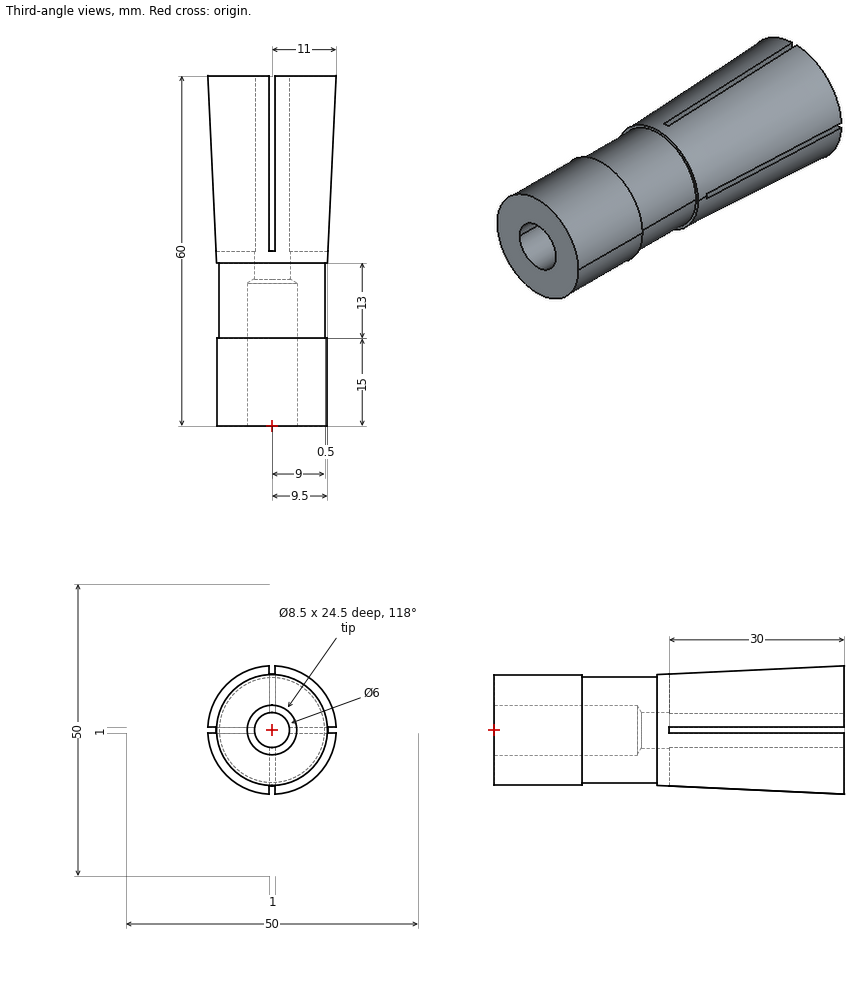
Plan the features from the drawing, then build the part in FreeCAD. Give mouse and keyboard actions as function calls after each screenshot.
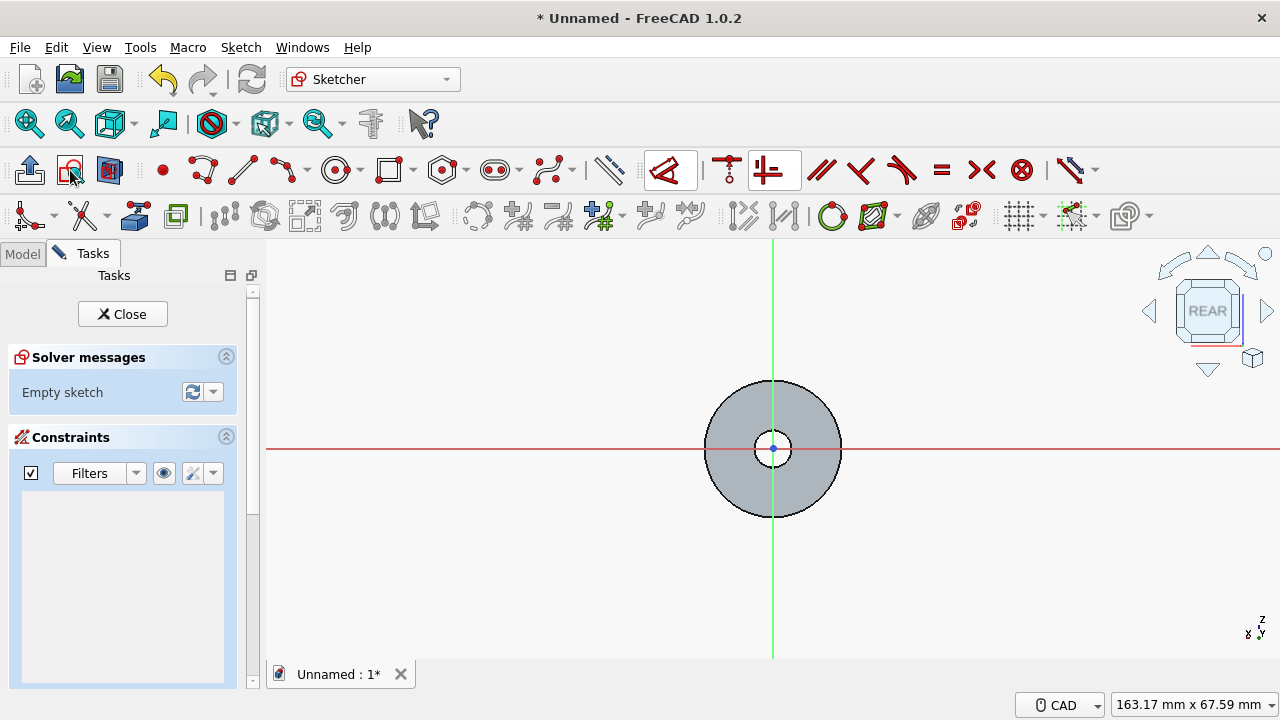
scroll(856, 449, up, 3)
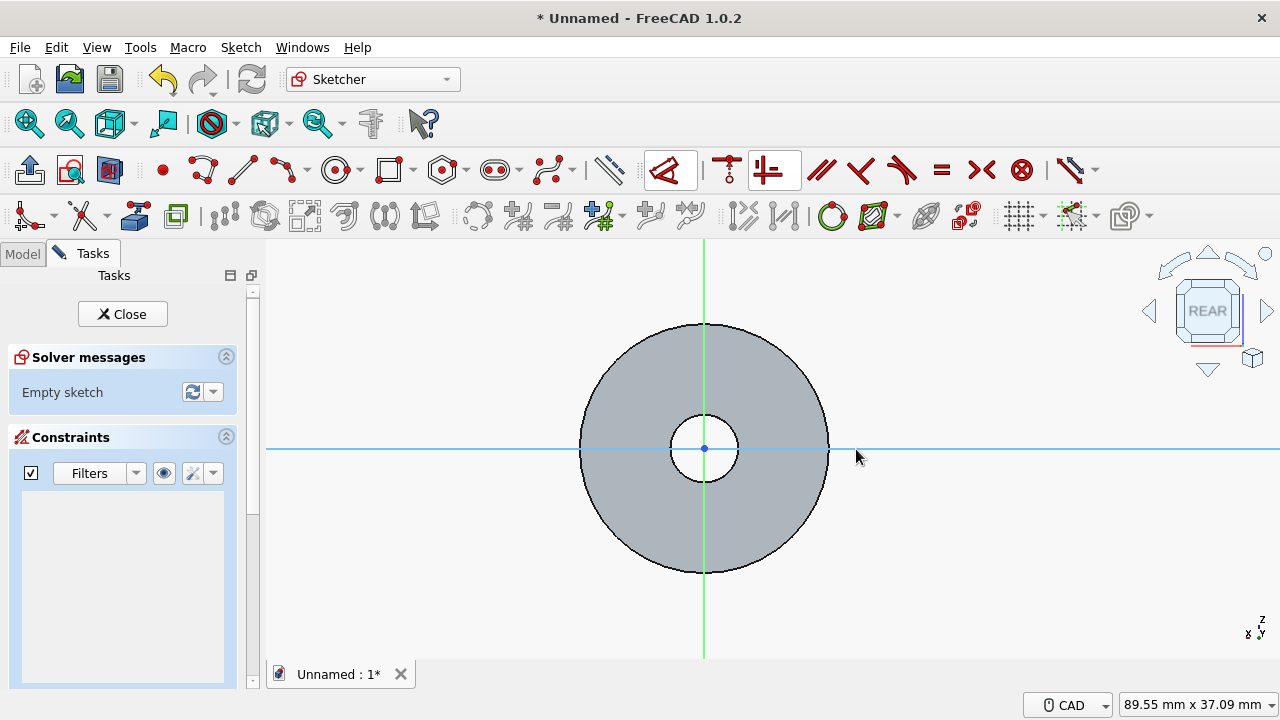
key(g)
key(v)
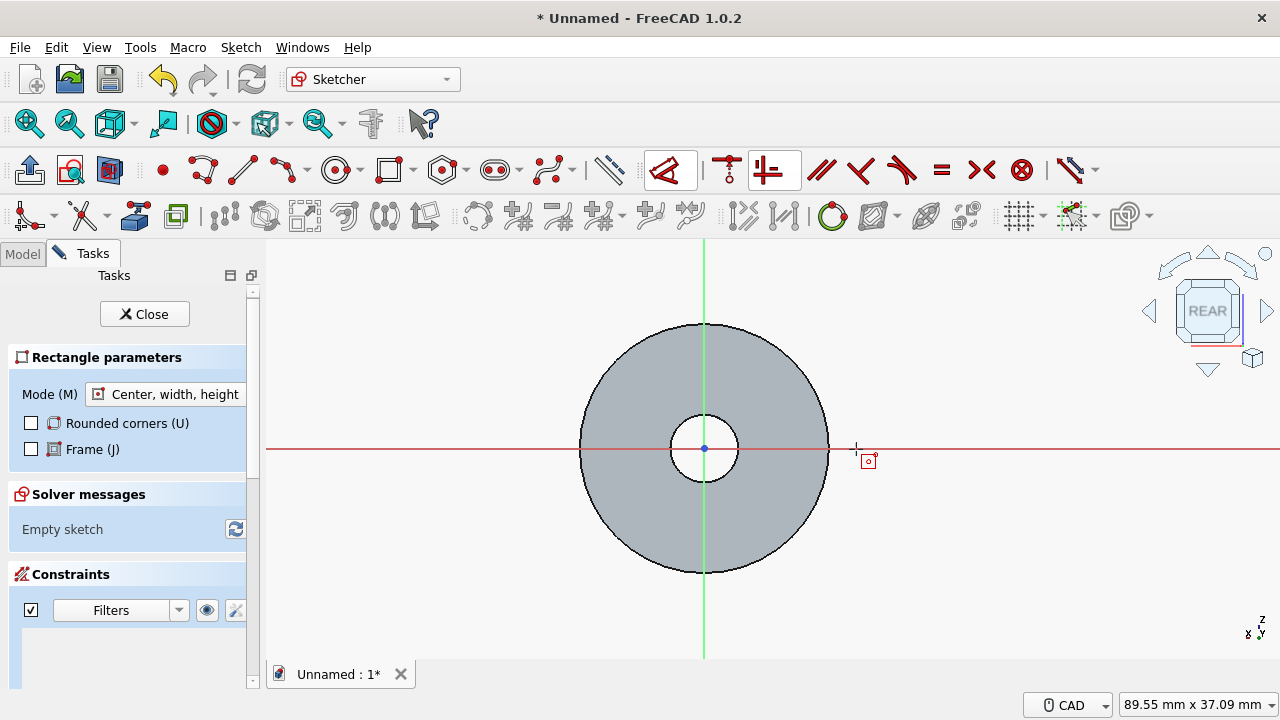
scroll(704, 449, up, 6)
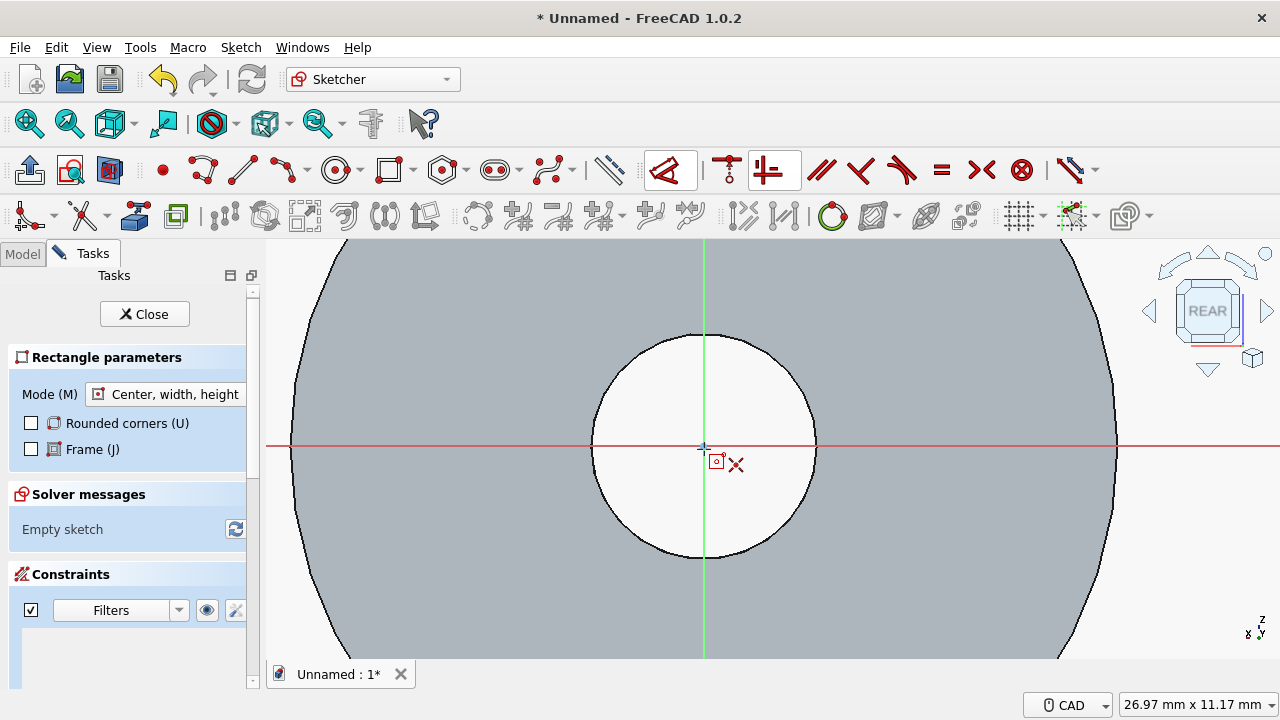
click(704, 446)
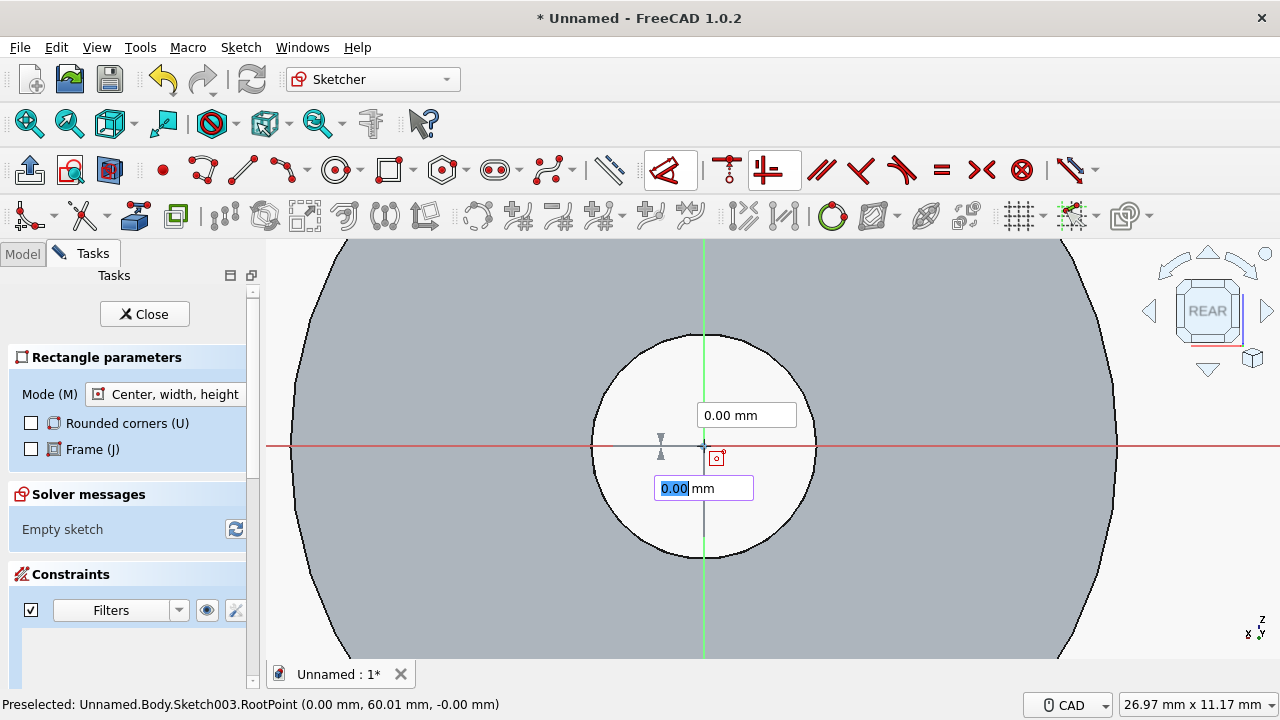
scroll(705, 450, down, 6)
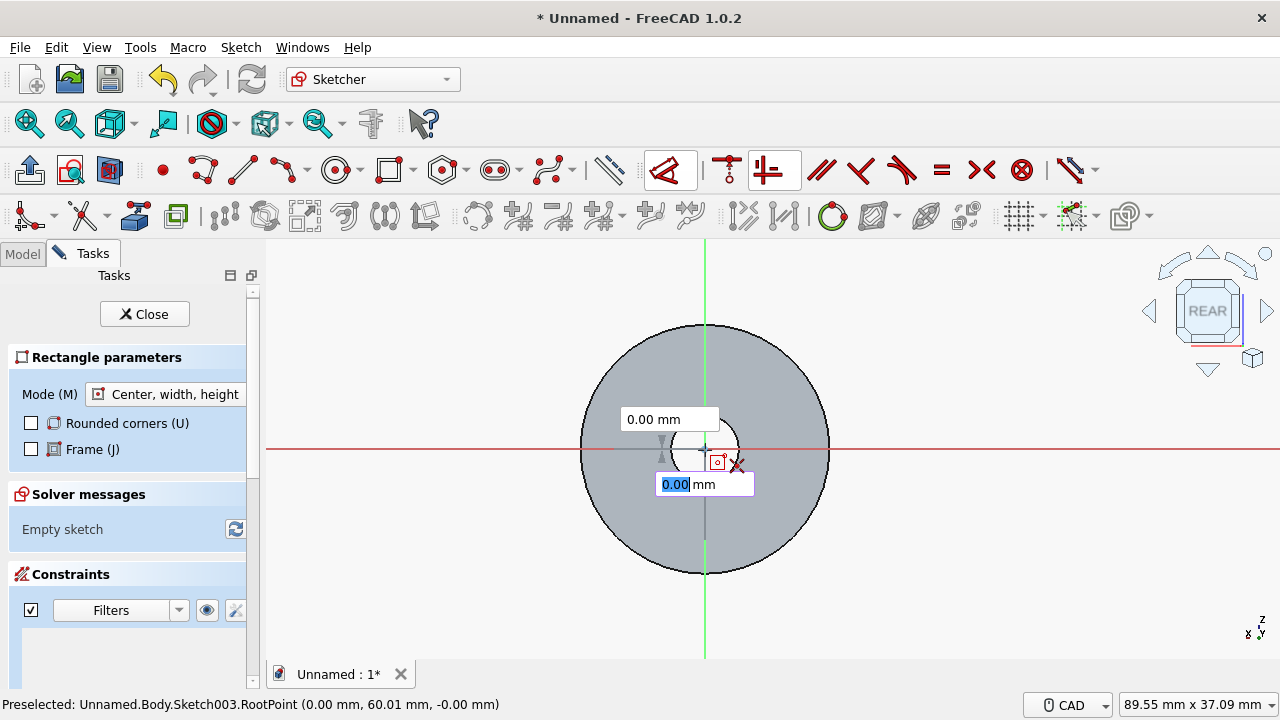
scroll(988, 444, up, 6)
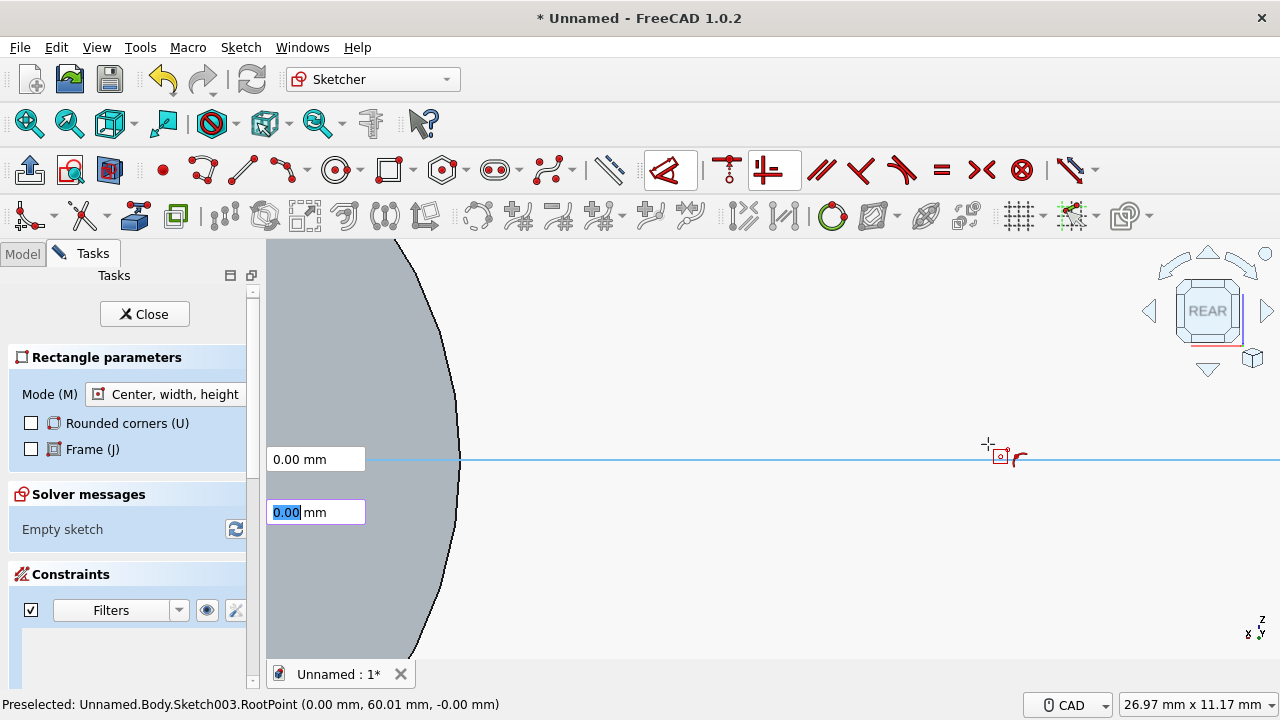
click(987, 442)
key(Escape)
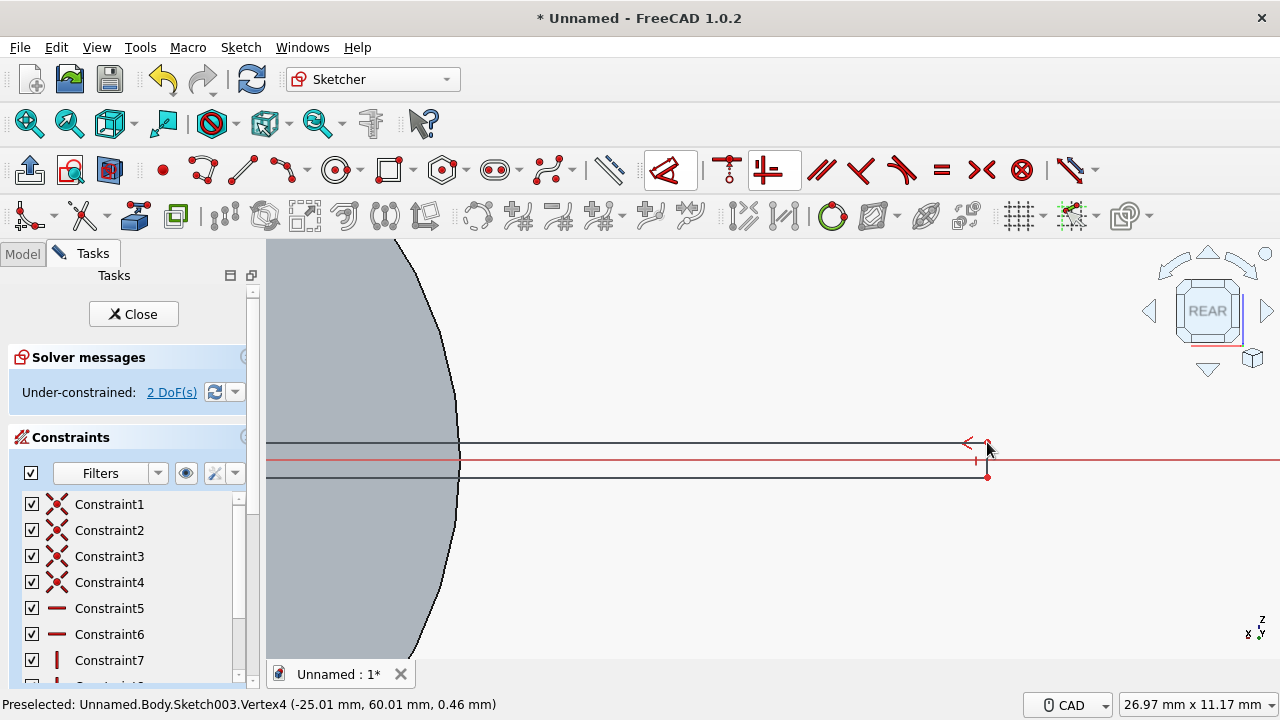
click(987, 464)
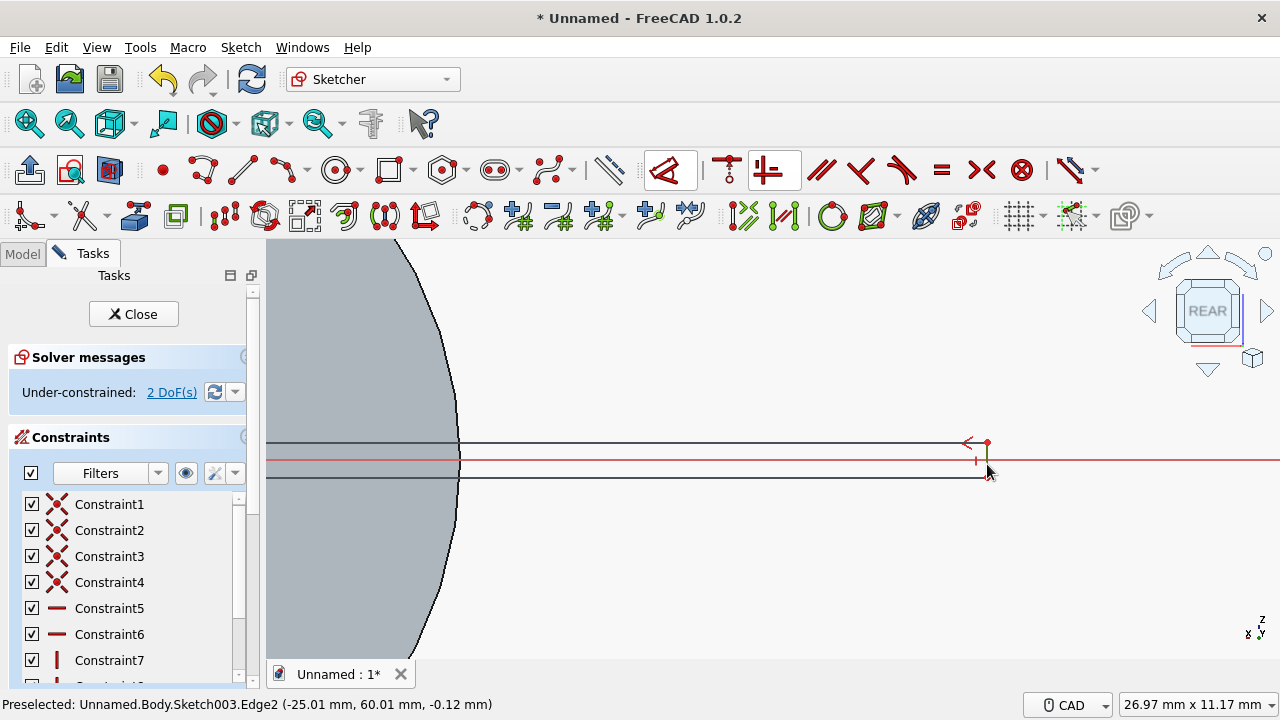
key(i)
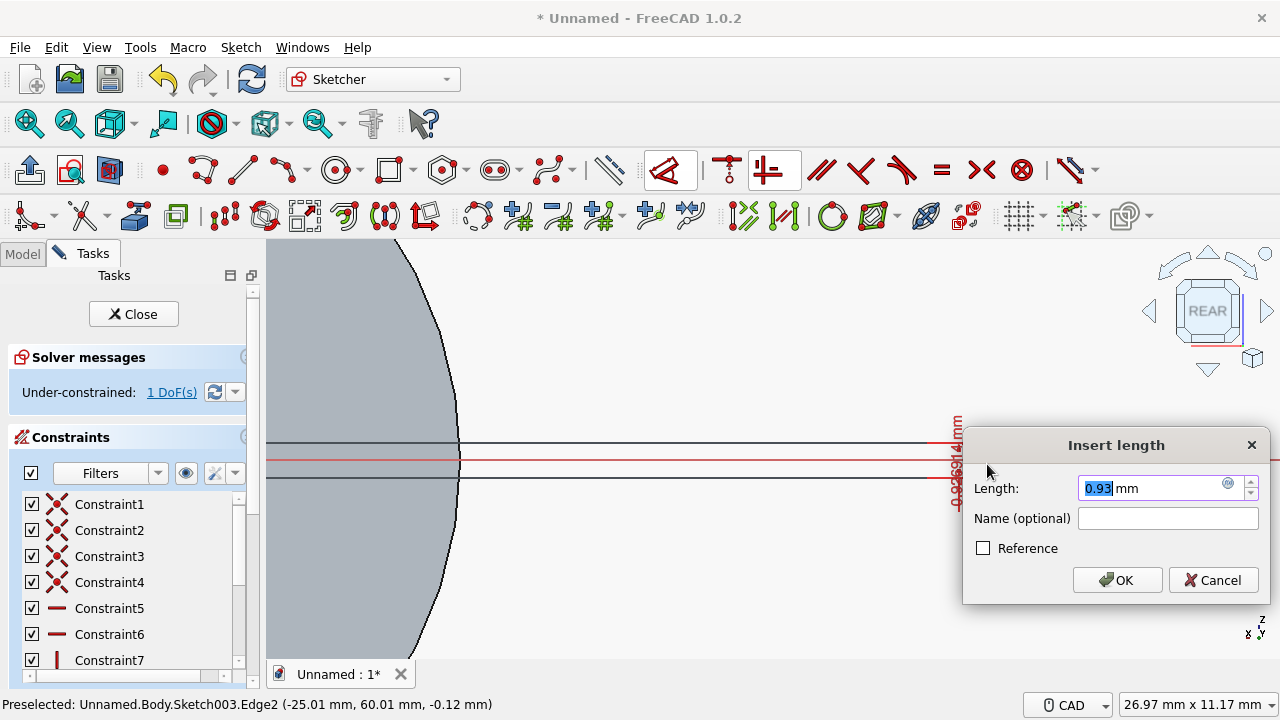
text(1)
key(Return)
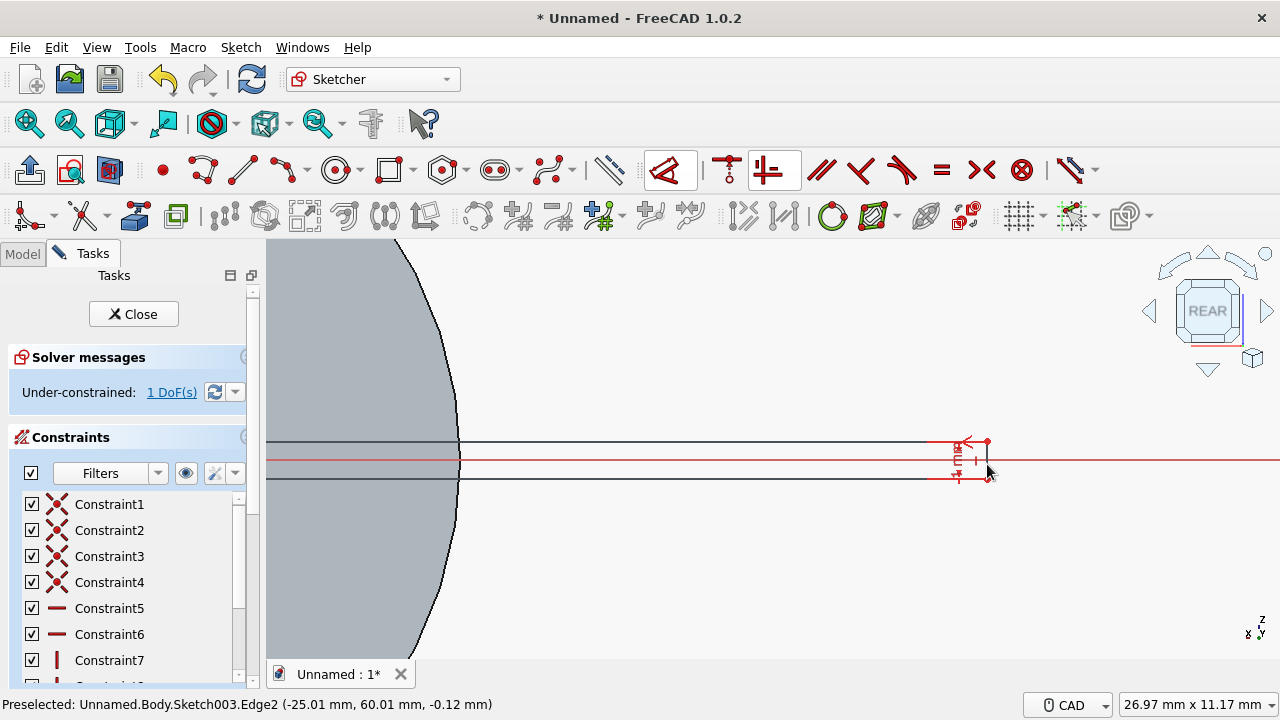
click(423, 479)